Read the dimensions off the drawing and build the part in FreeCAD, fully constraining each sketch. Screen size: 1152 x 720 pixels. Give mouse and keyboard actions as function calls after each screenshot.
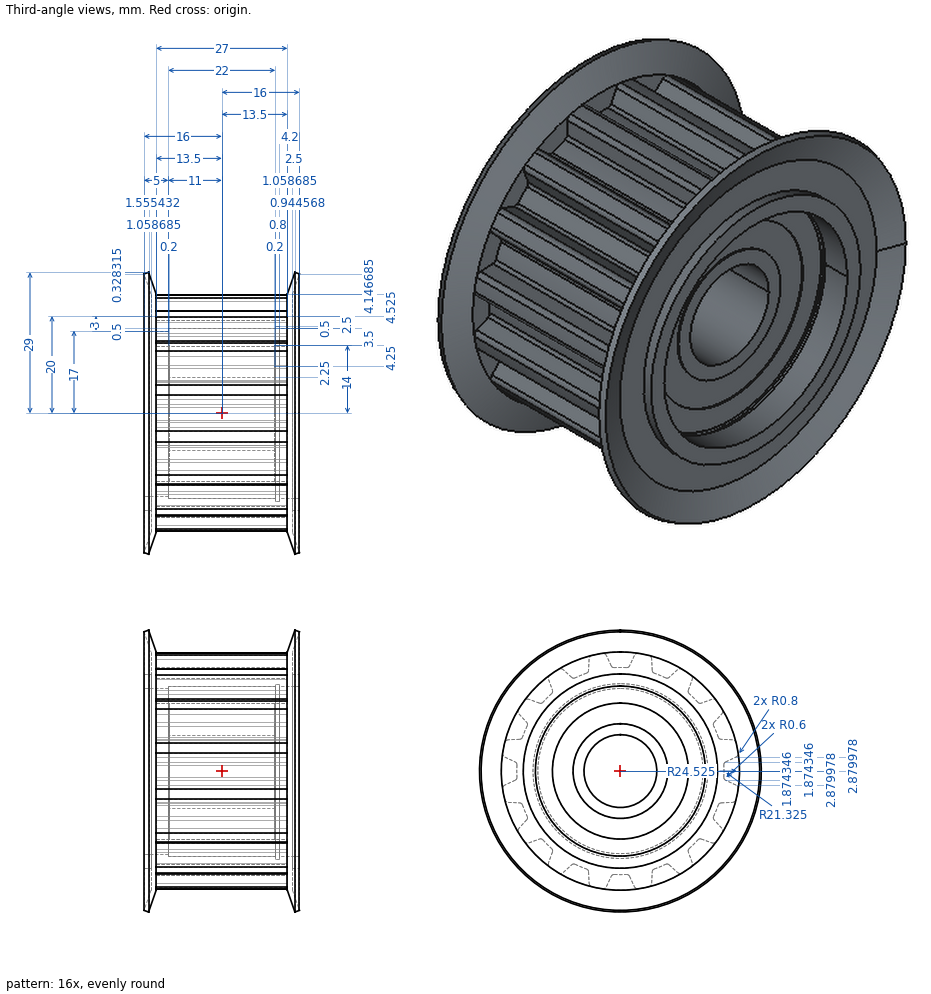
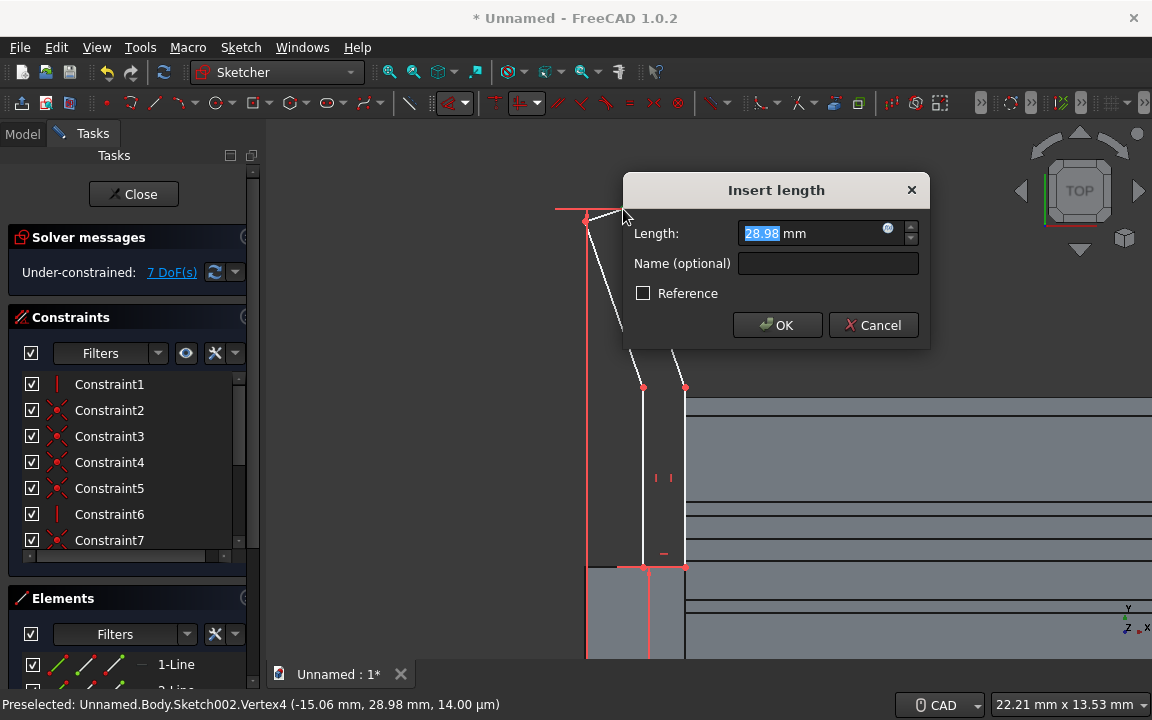
text(29)
key(Return)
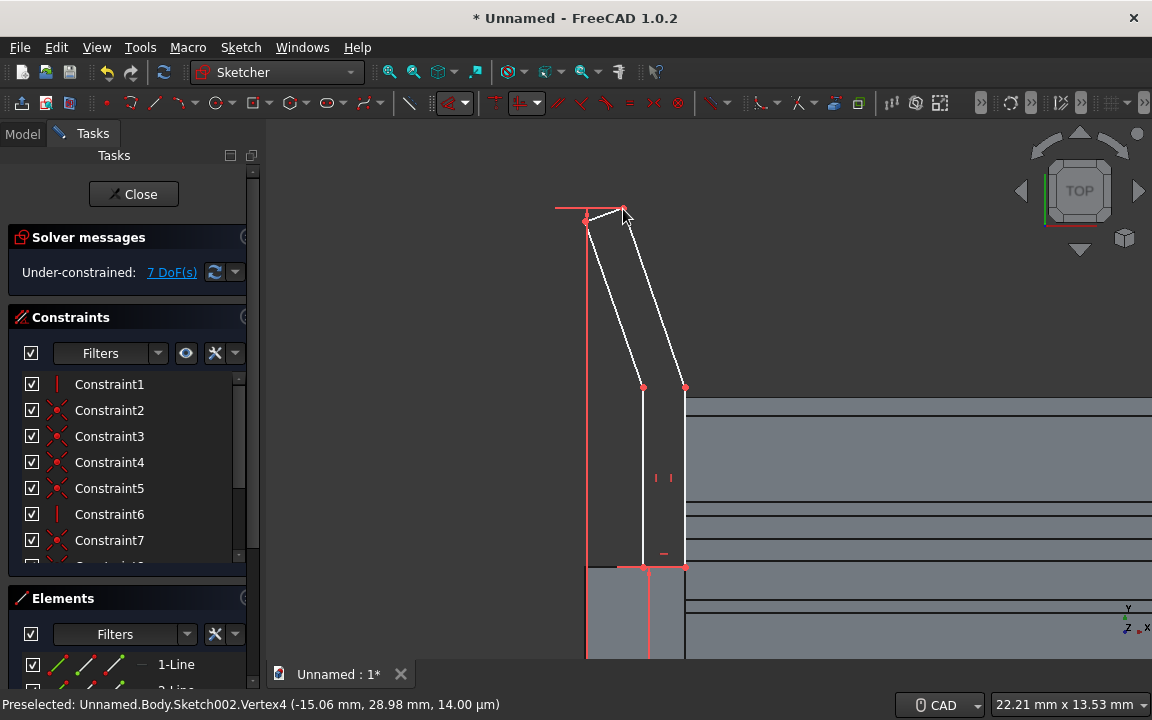
click(585, 222)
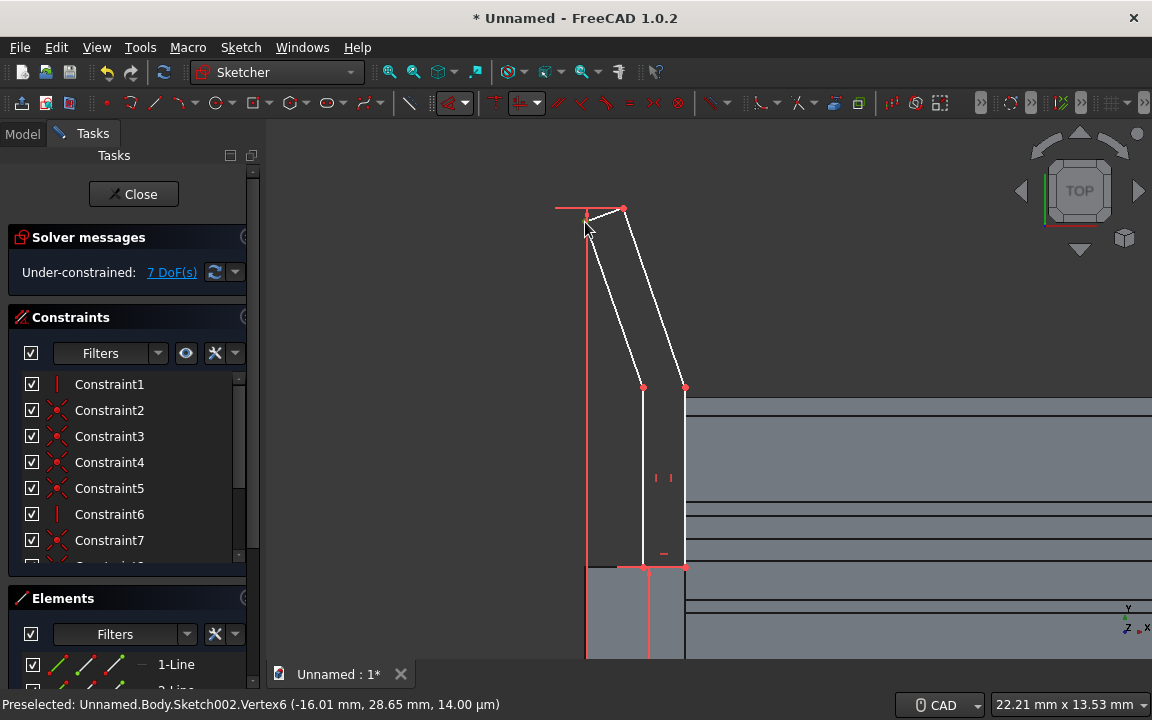
click(468, 104)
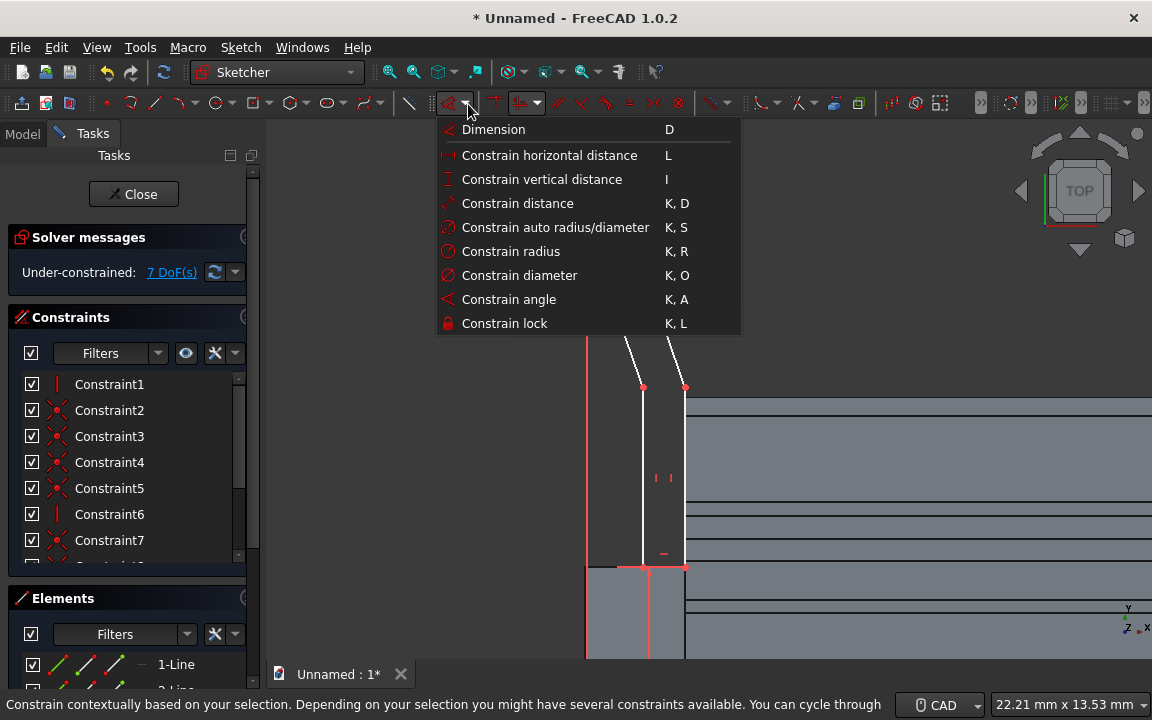
click(589, 155)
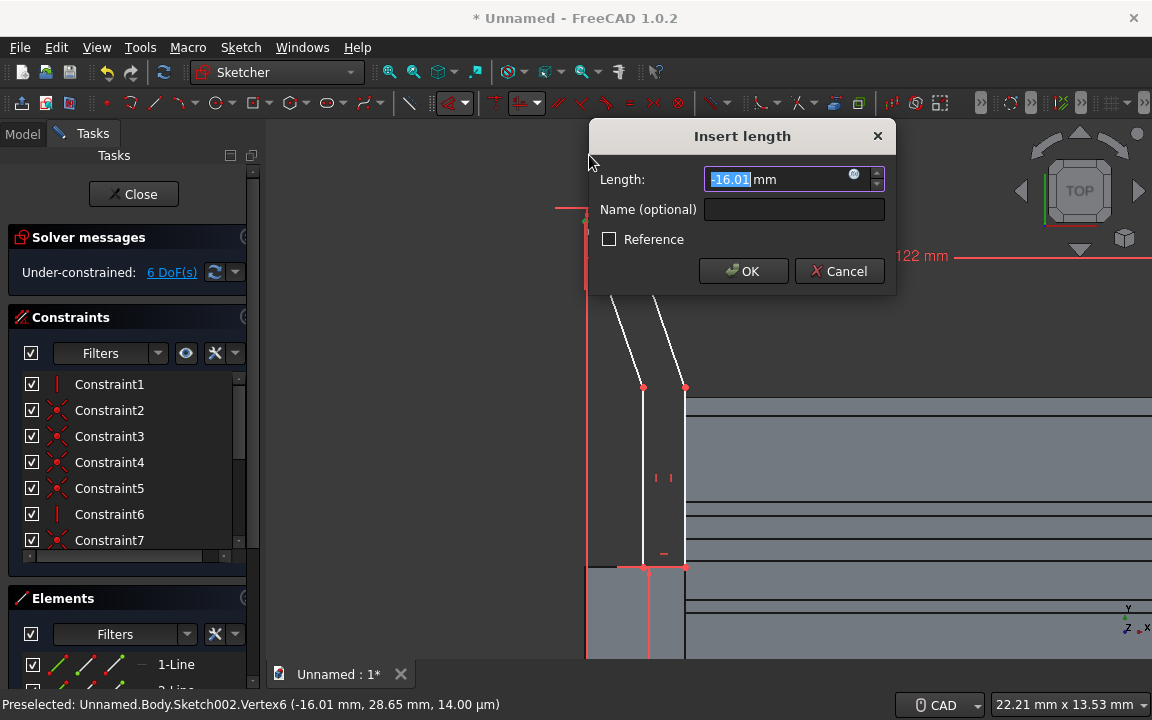
text(-16)
key(Return)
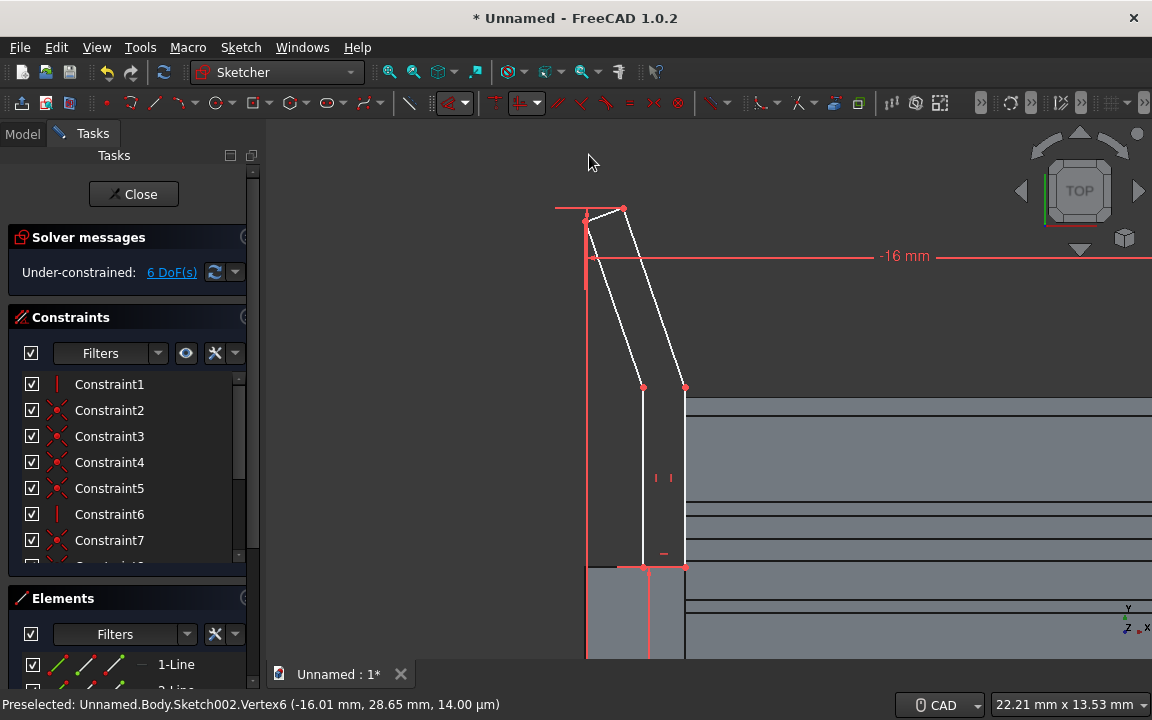
click(685, 513)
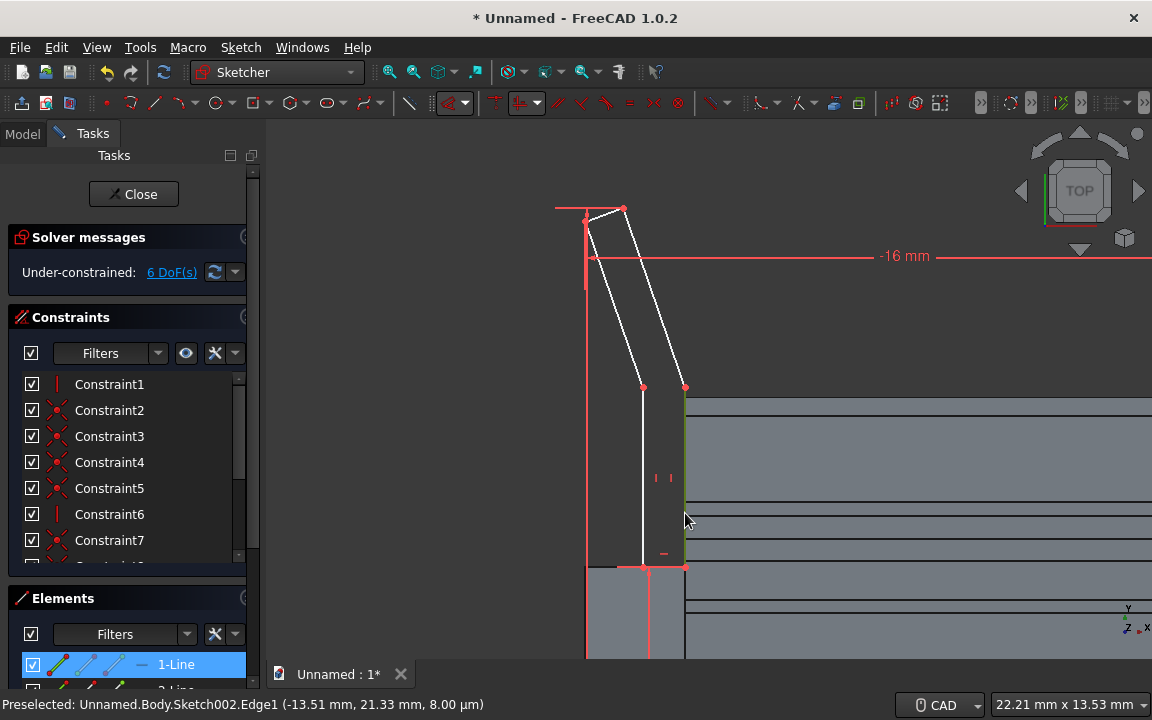
click(468, 104)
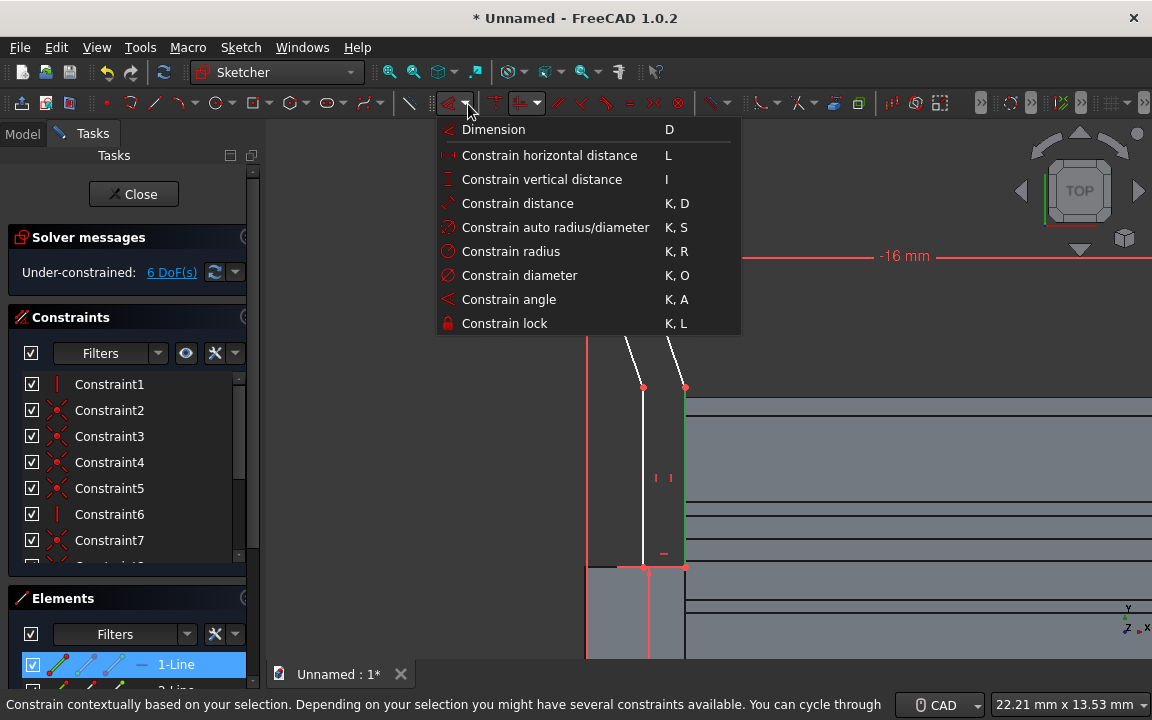
click(589, 179)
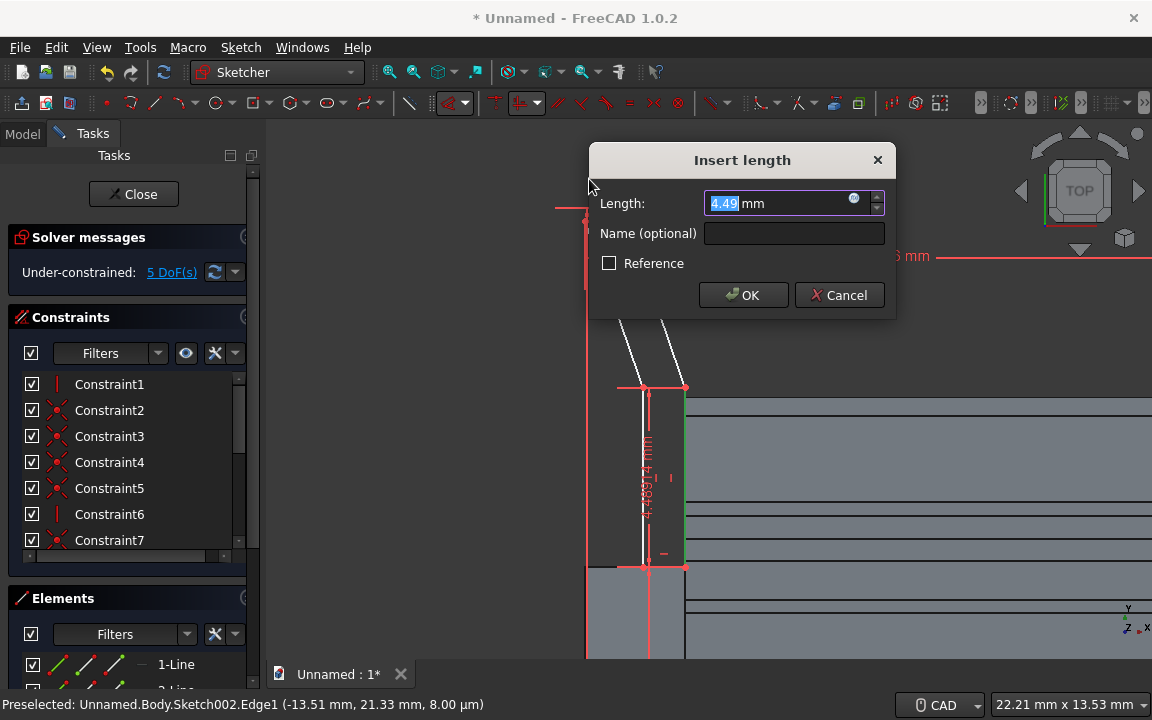
text(4.525)
key(Return)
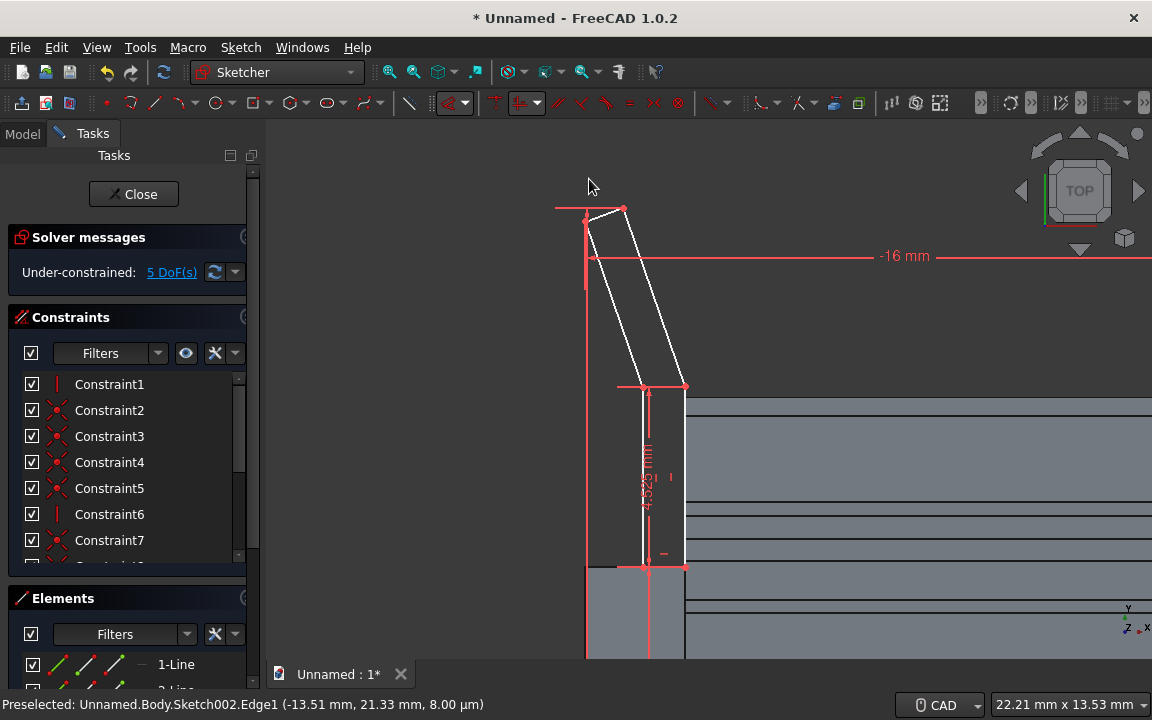
click(643, 442)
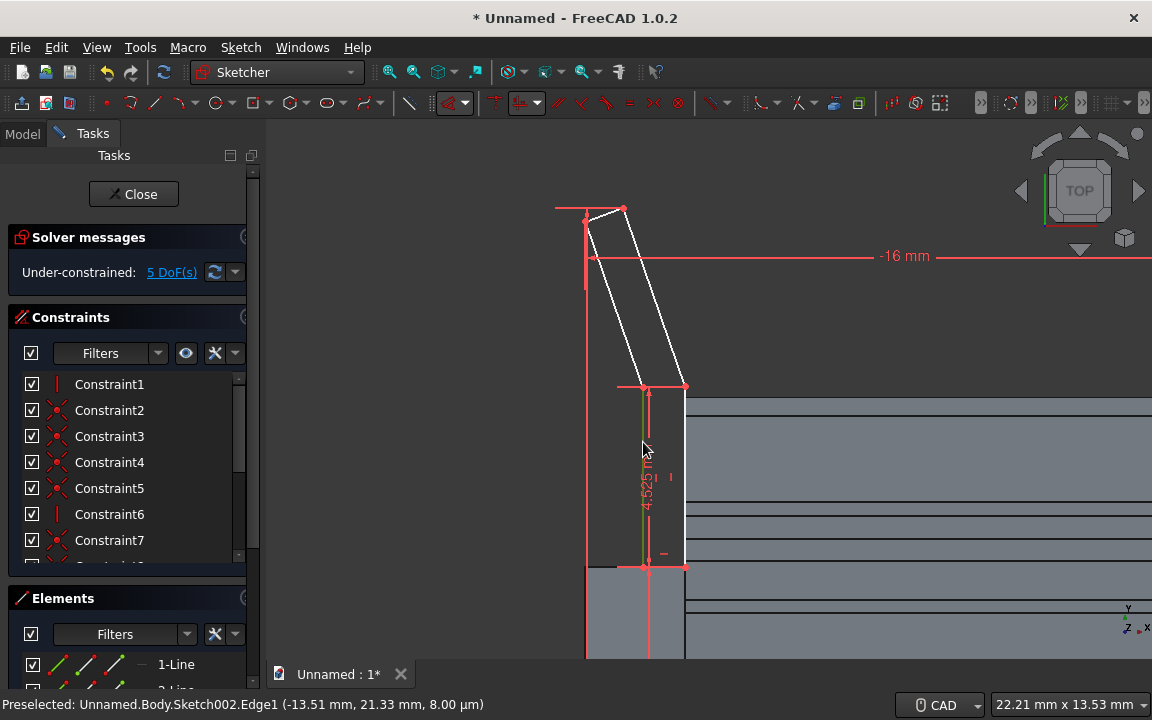
key(i)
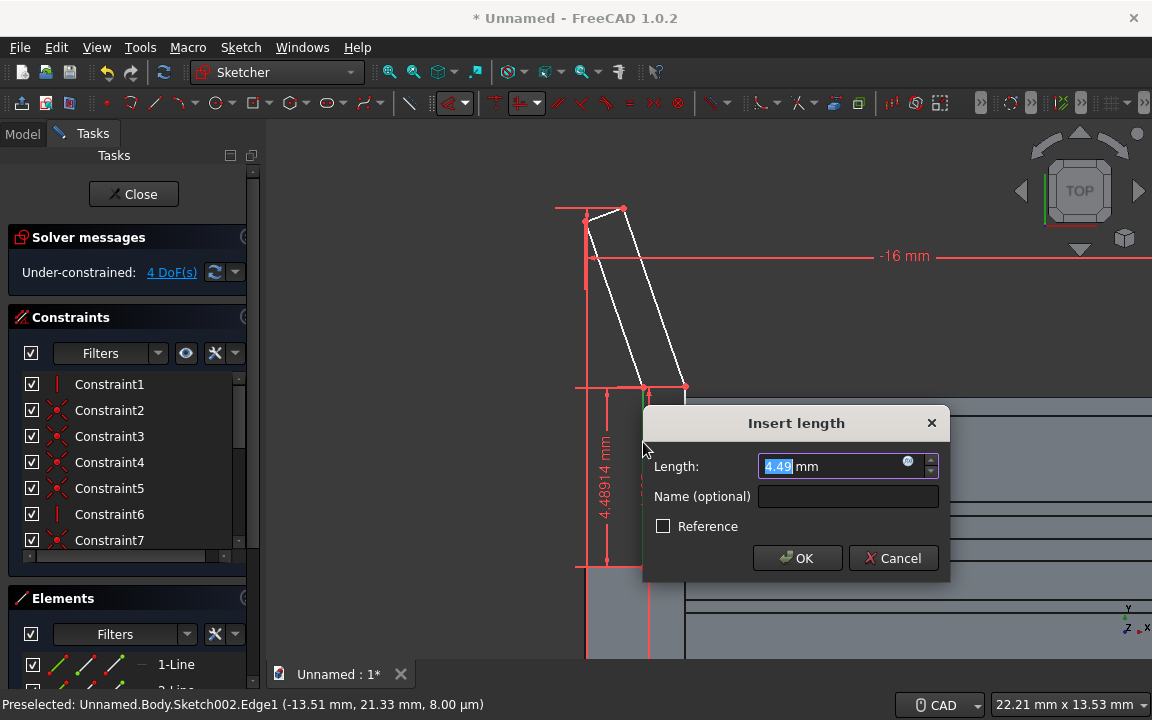
text(4.525)
key(Return)